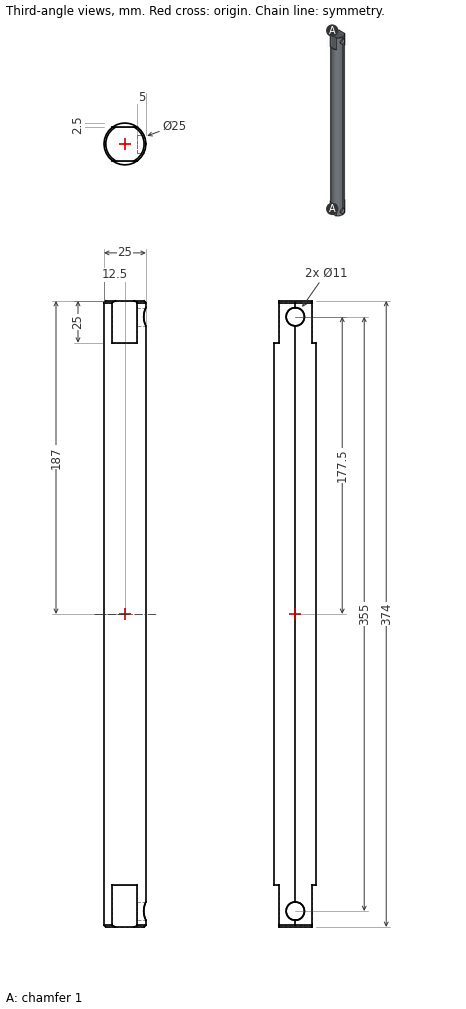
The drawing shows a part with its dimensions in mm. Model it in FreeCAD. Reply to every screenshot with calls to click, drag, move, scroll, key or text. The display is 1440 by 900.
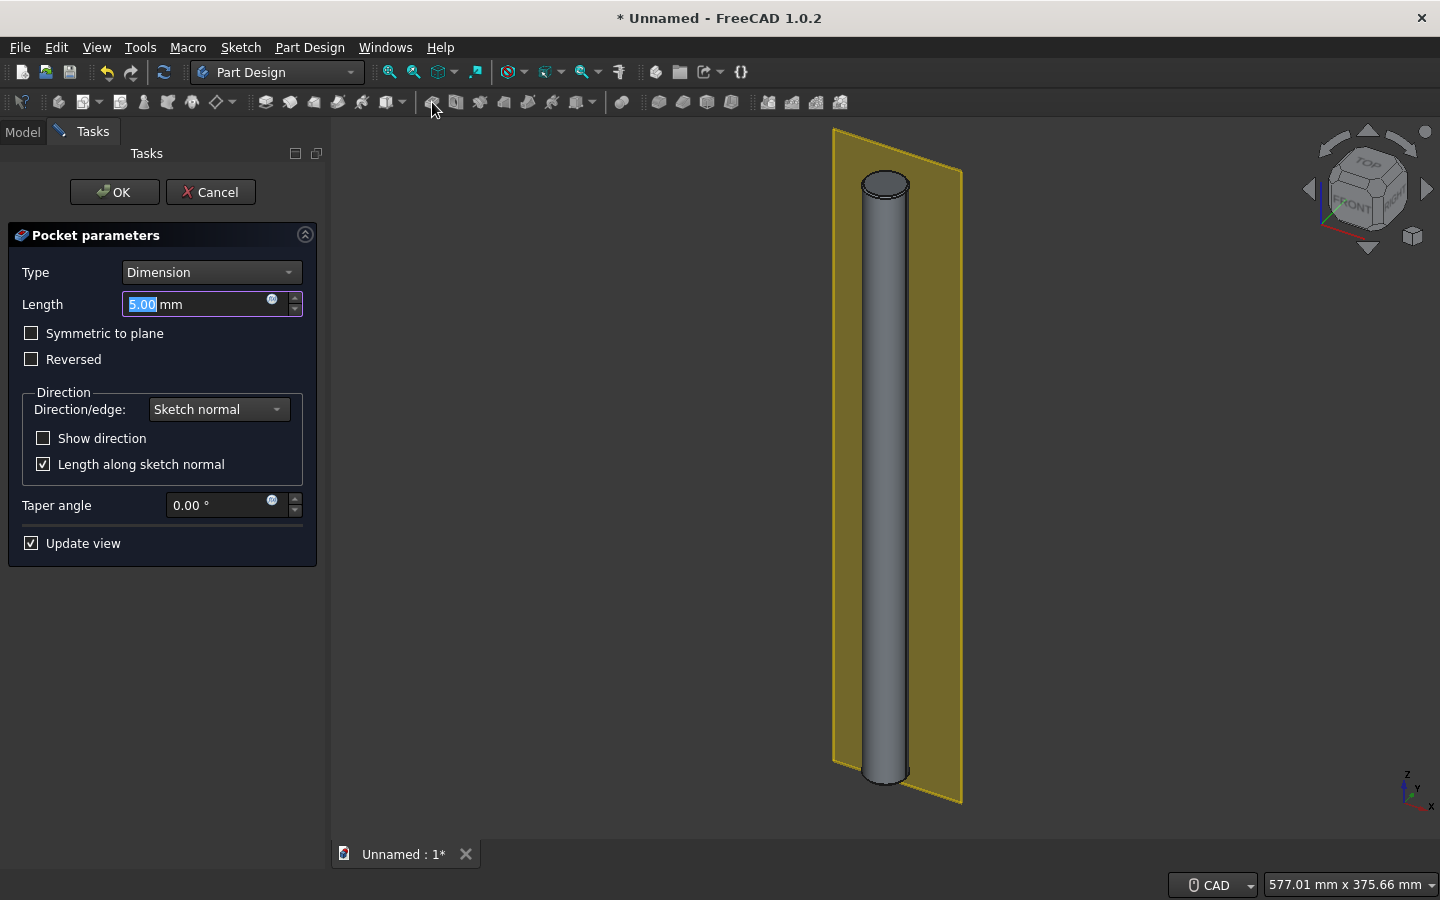
text(2.5)
key(Tab)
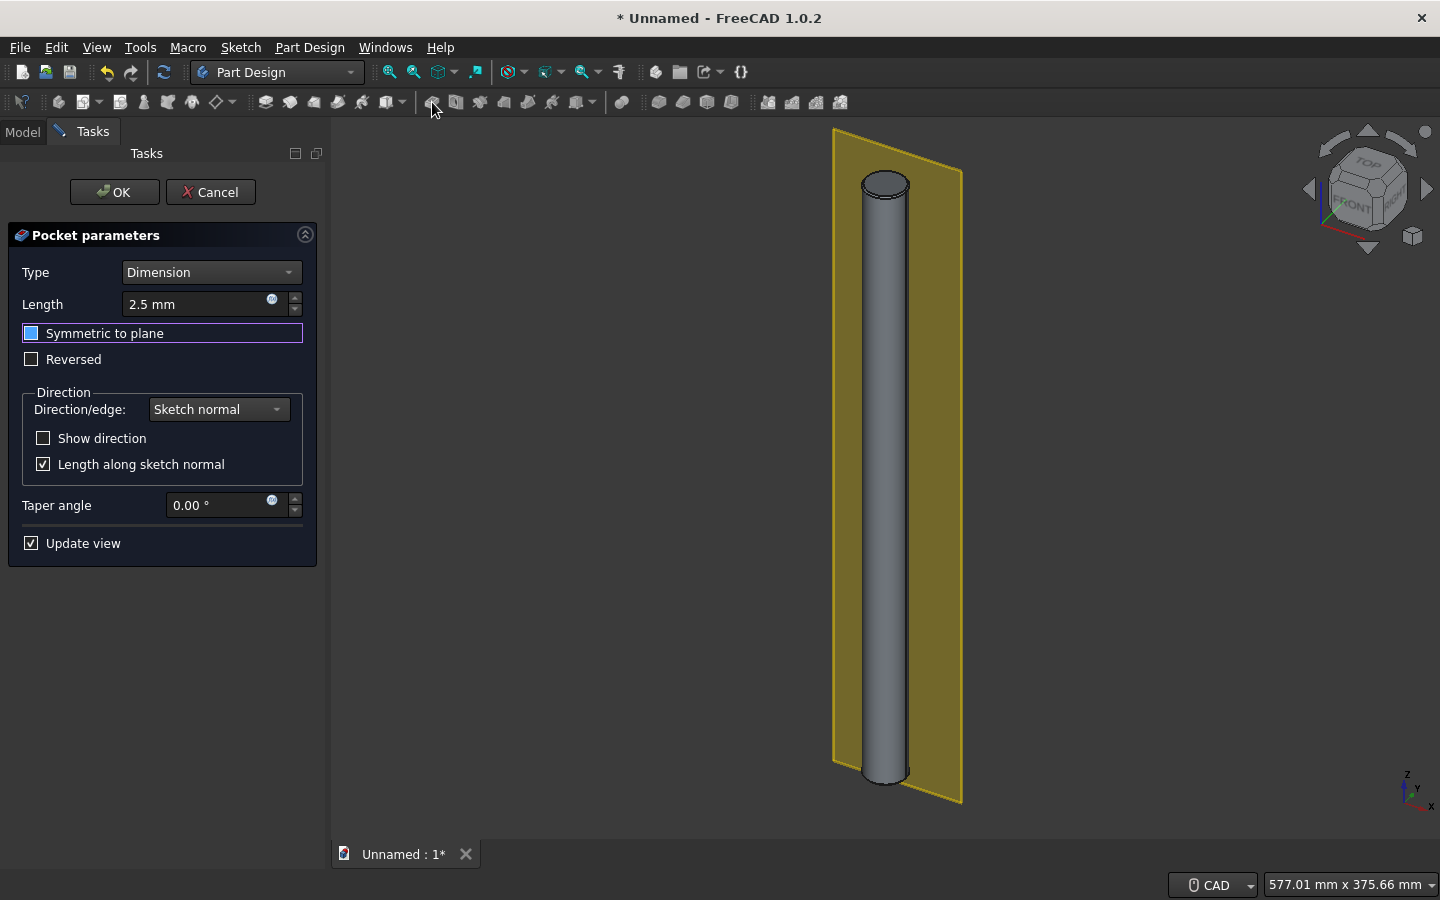
click(30, 359)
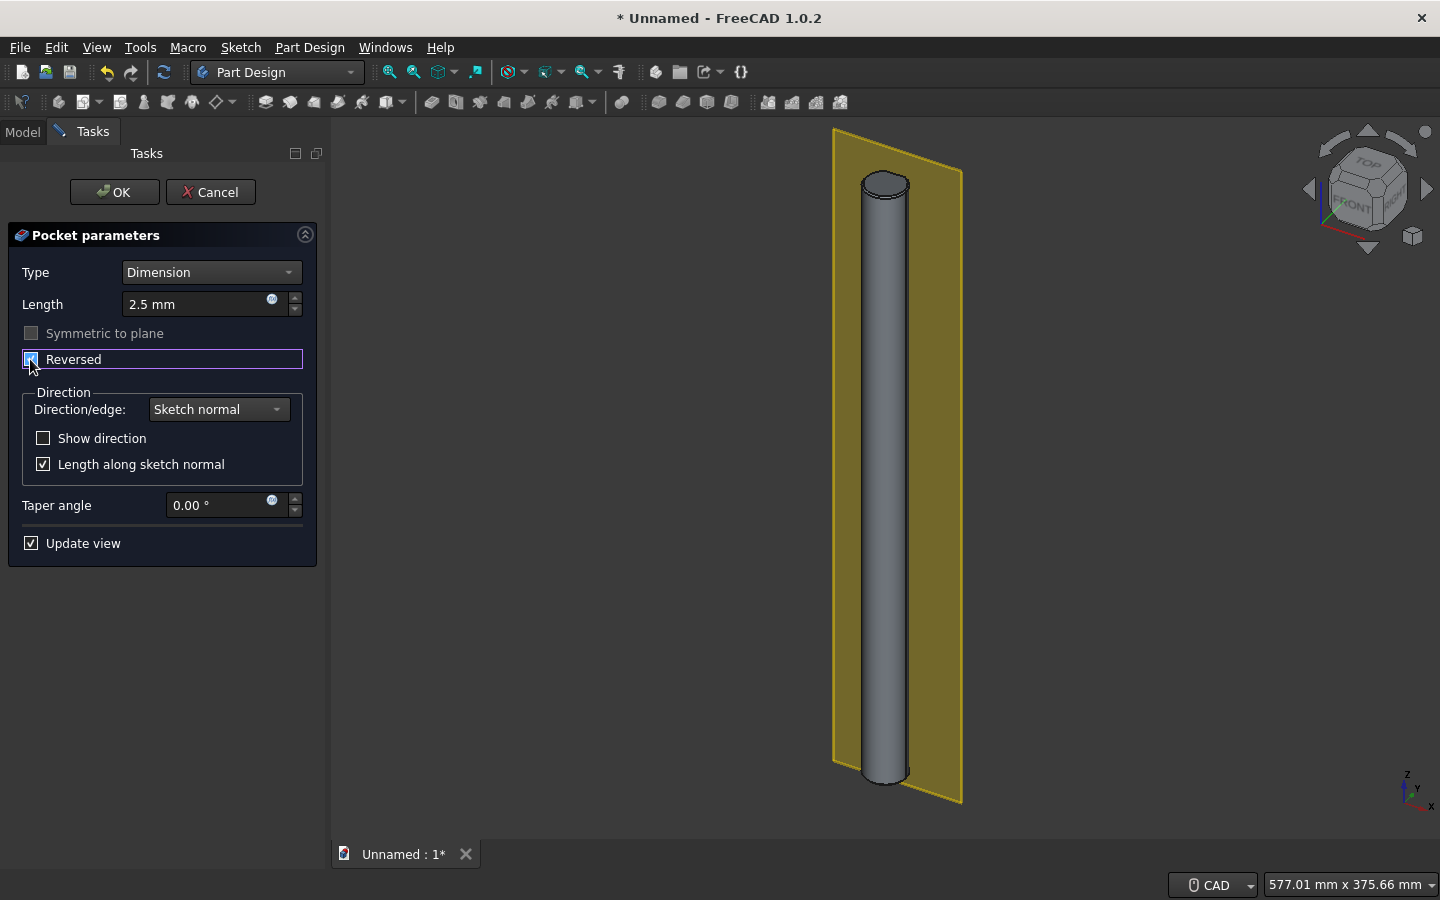
click(115, 192)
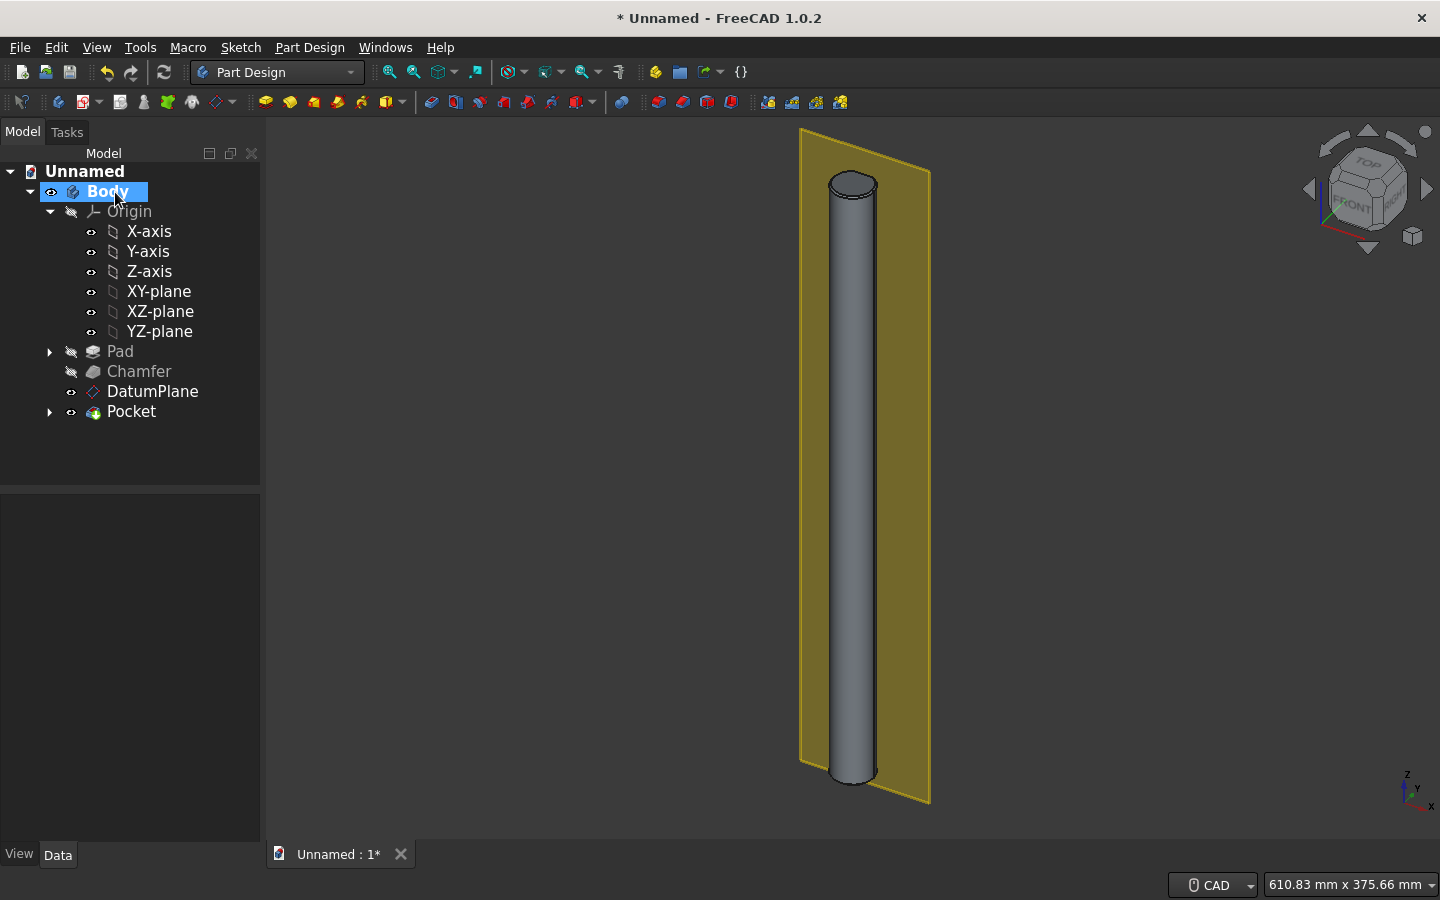
click(116, 392)
key(space)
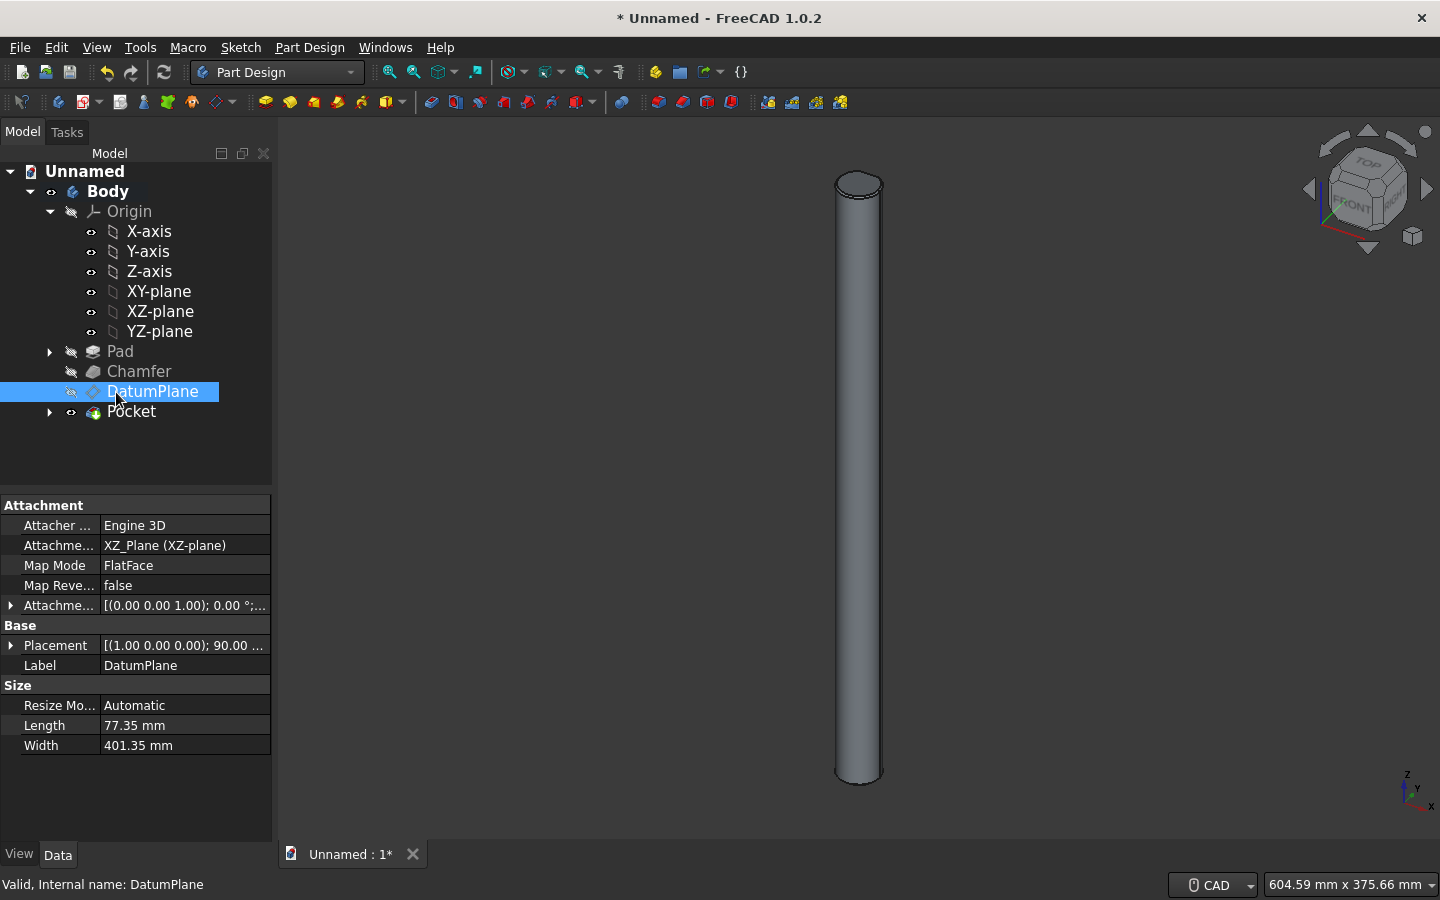
click(116, 412)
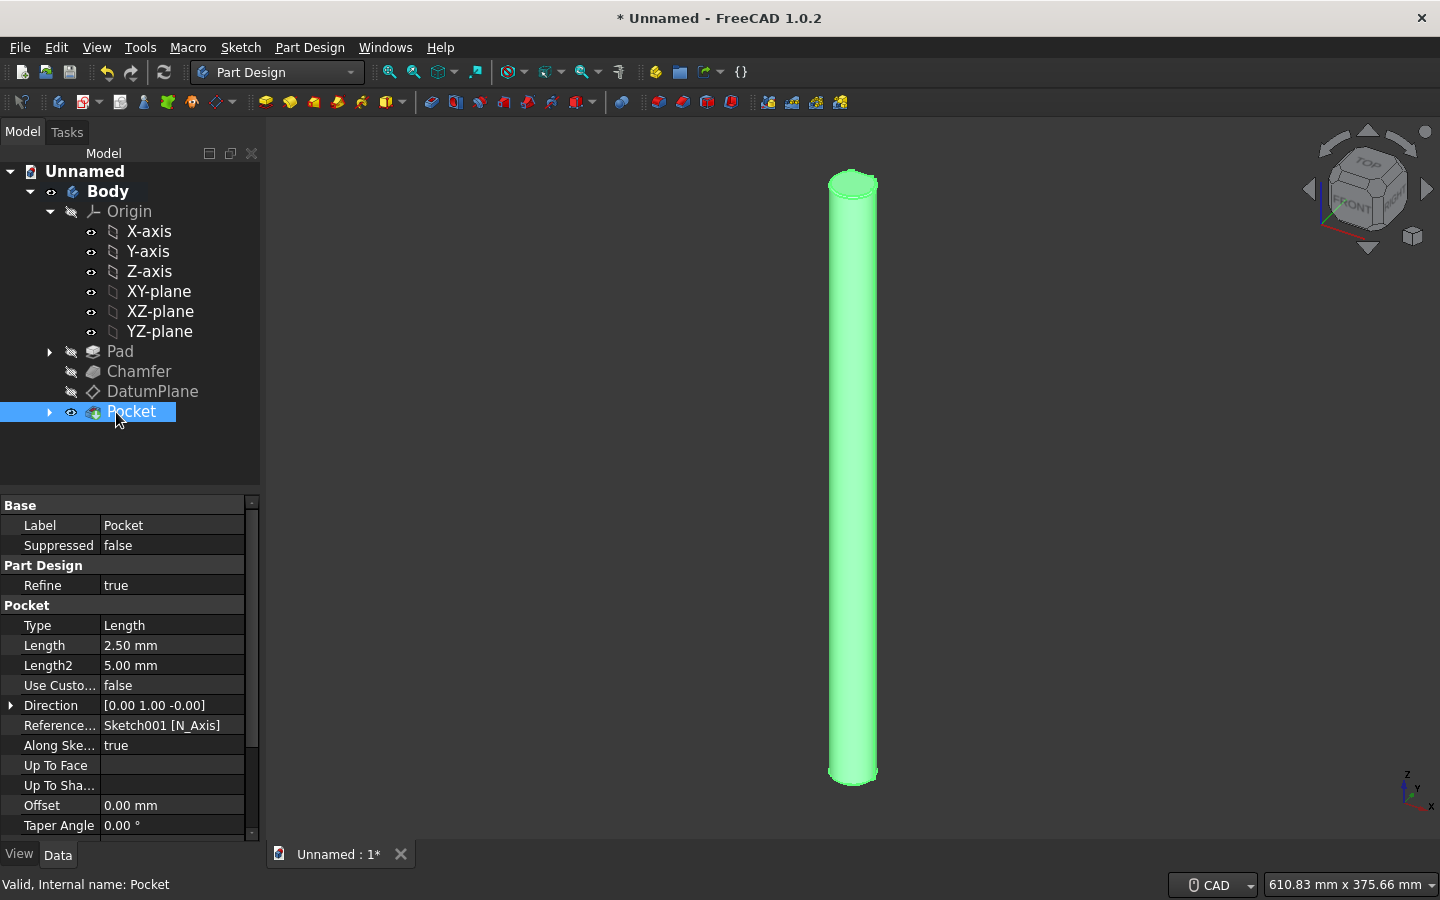
click(768, 102)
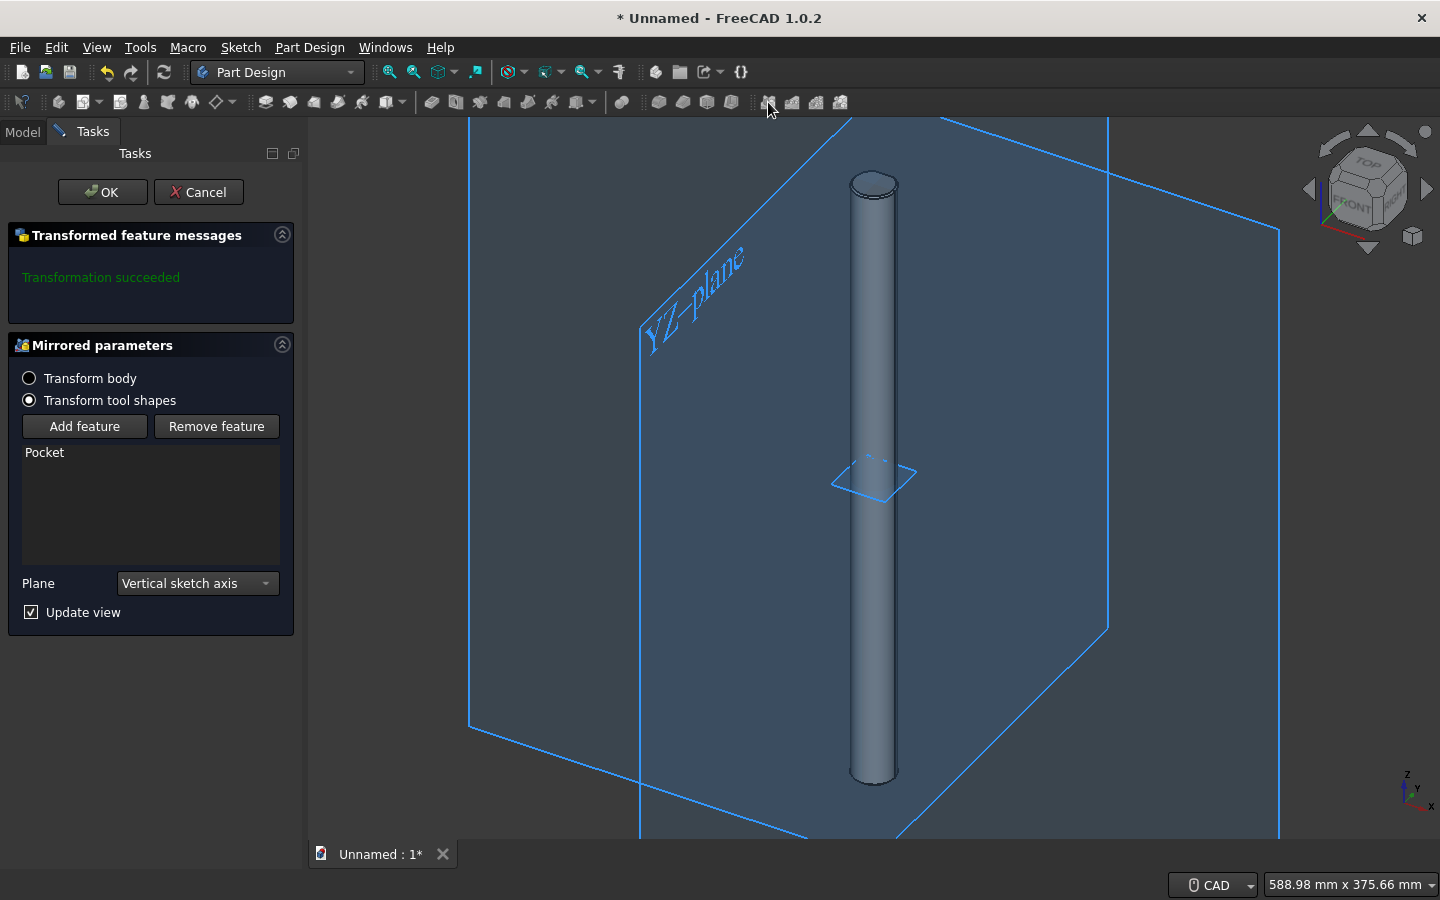
click(198, 584)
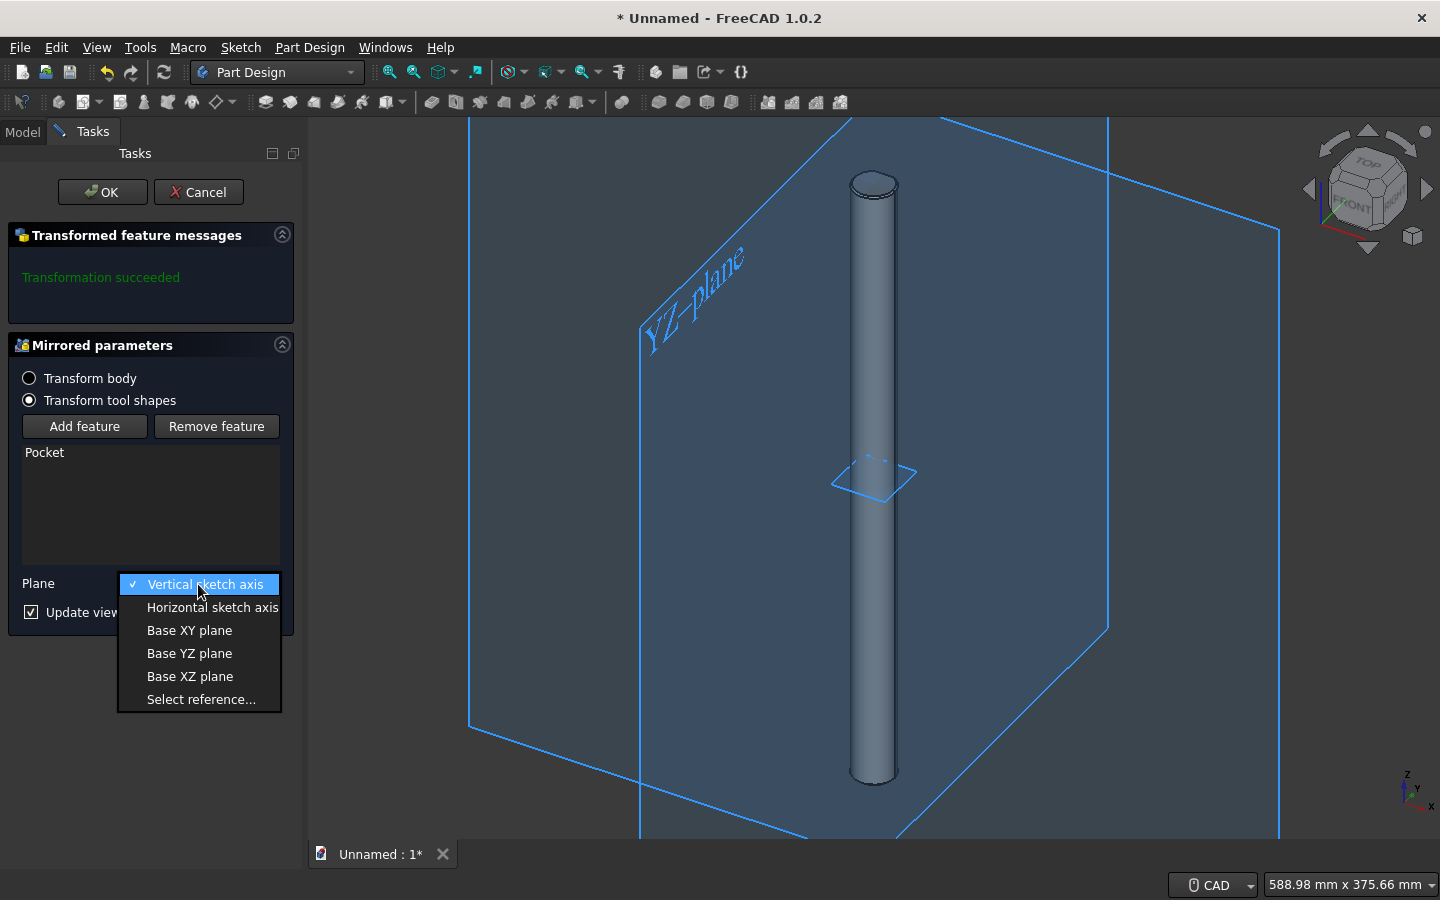
click(198, 676)